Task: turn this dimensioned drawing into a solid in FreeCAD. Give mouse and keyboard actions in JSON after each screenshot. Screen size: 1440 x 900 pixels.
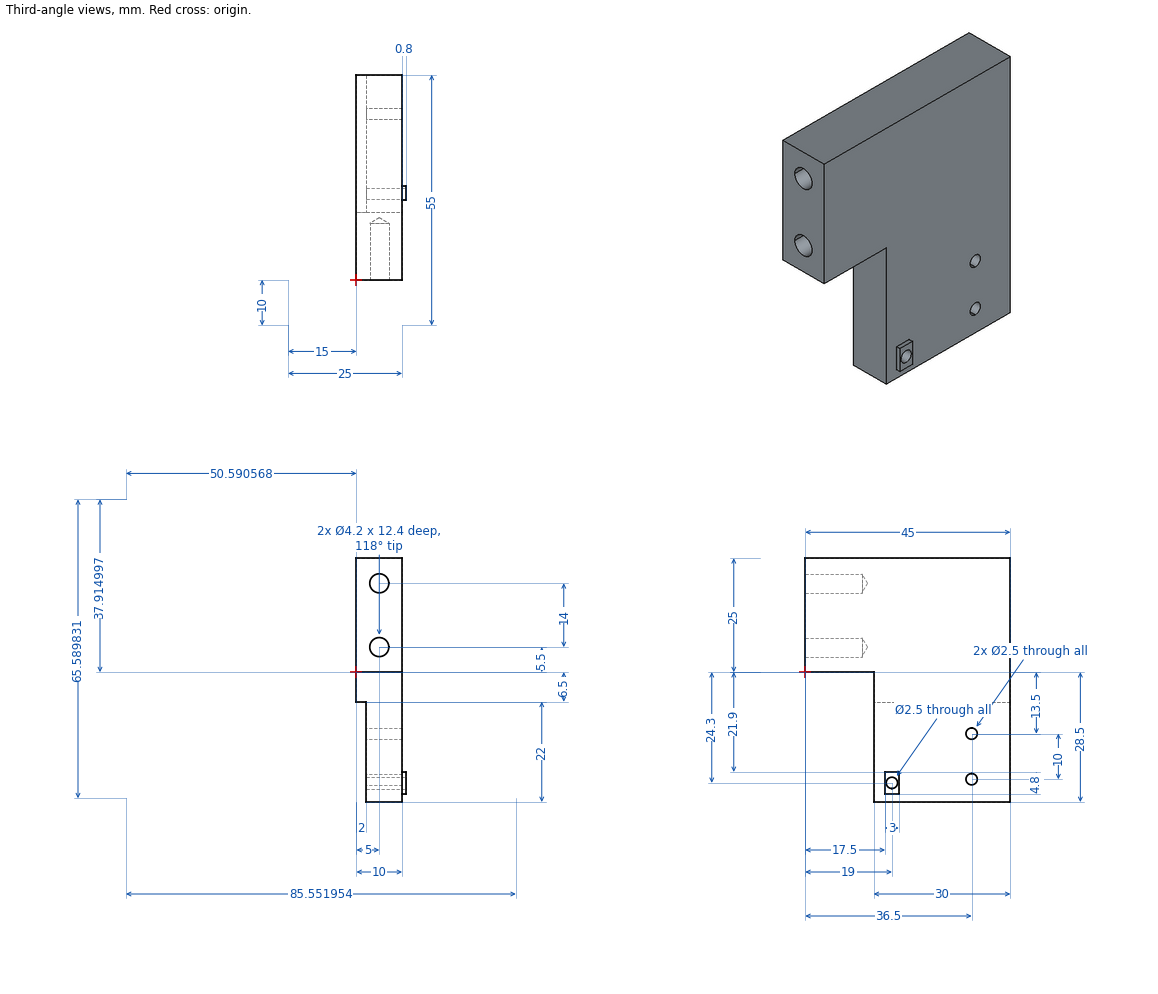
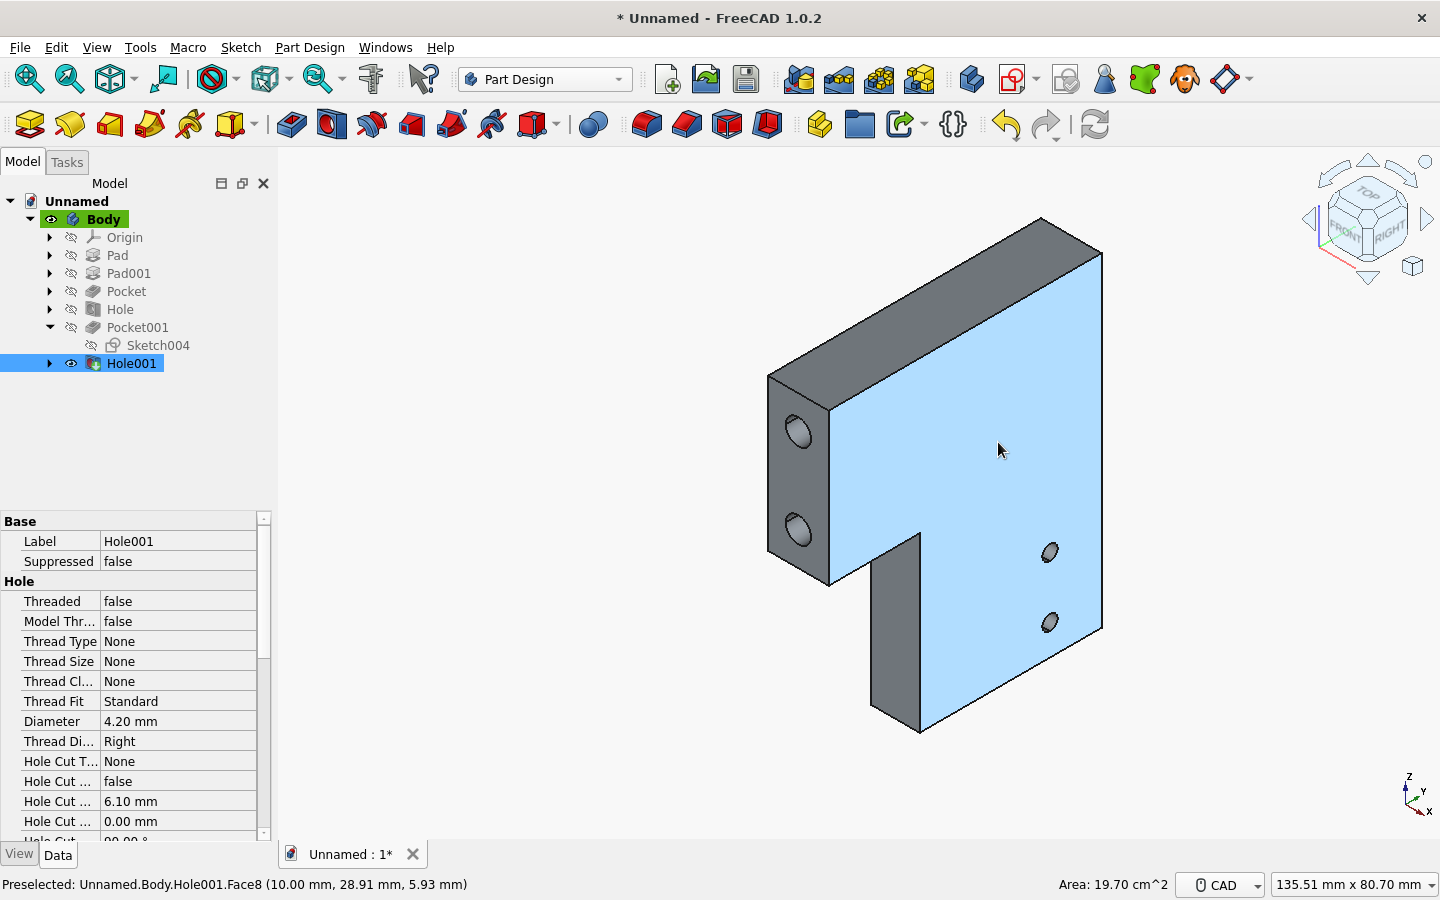
{"action": "left_click", "coordinate": [1012, 80]}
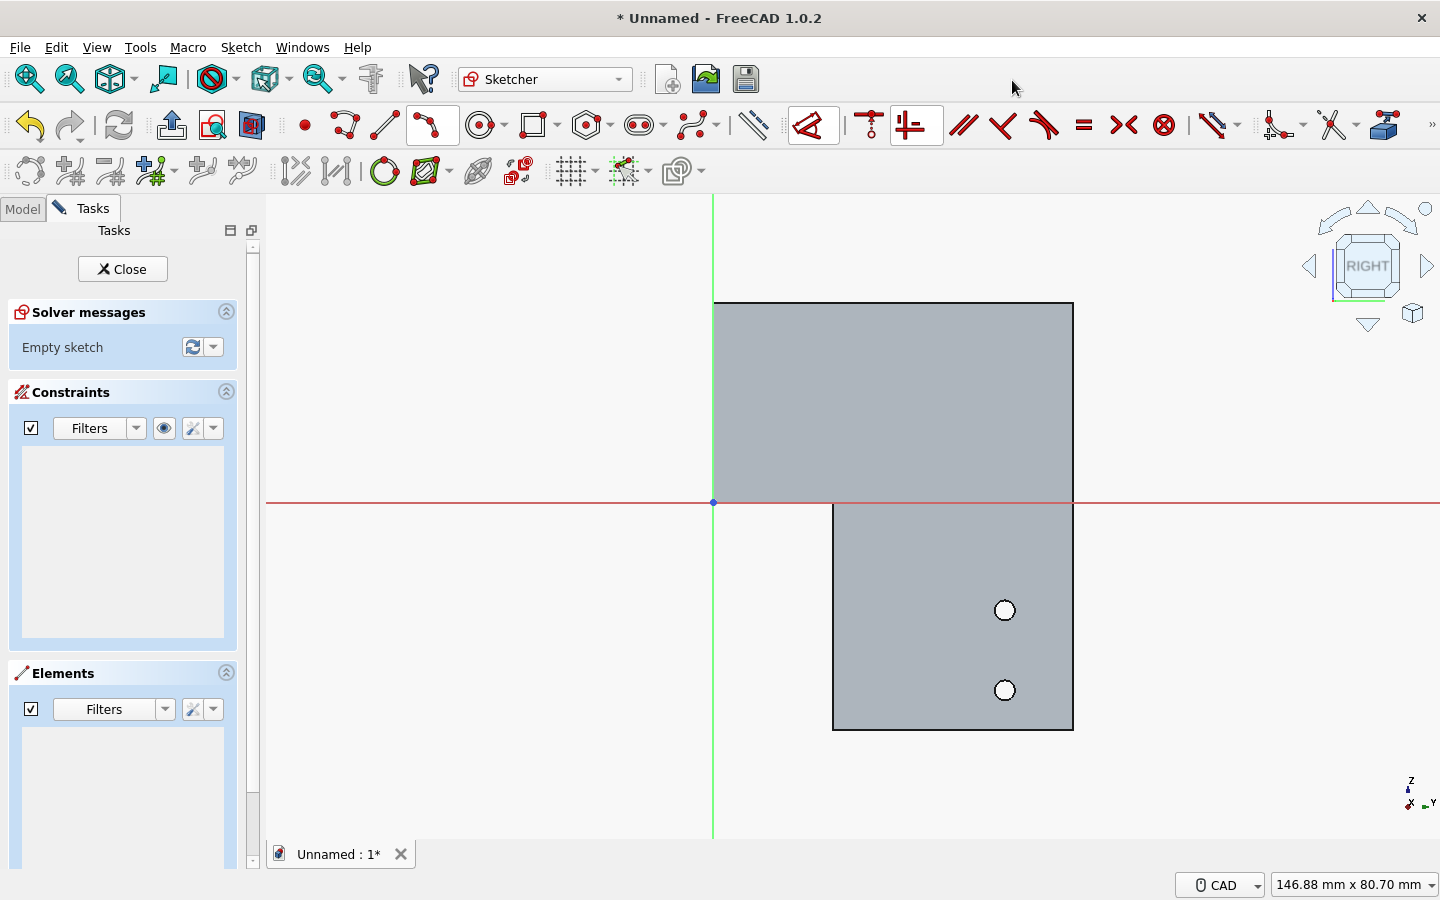
{"action": "scroll", "coordinate": [873, 715], "scroll_direction": "up", "scroll_amount": 12}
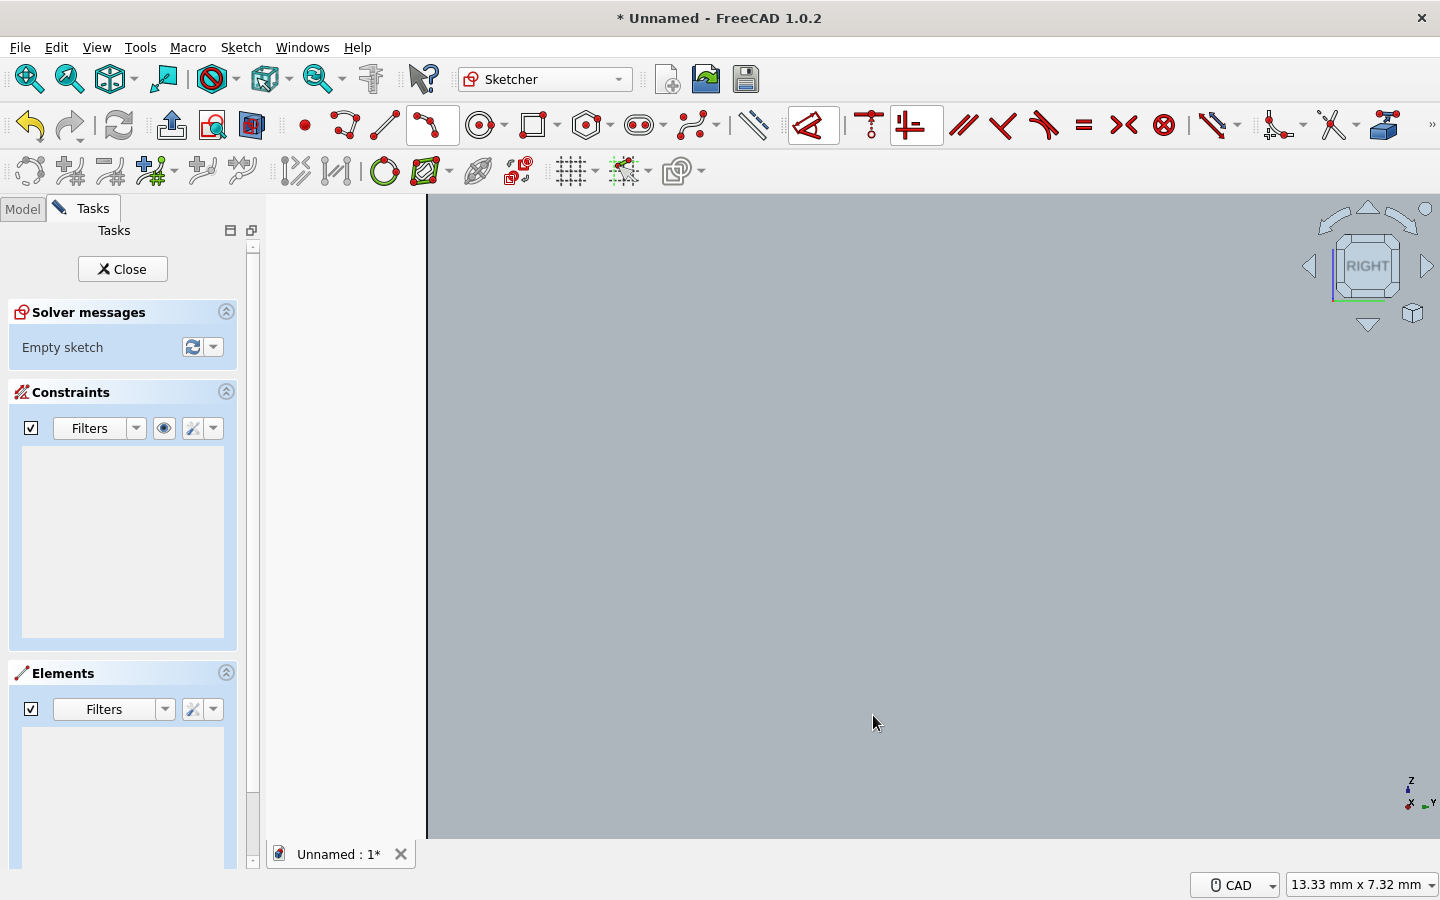
{"action": "left_click", "coordinate": [534, 126]}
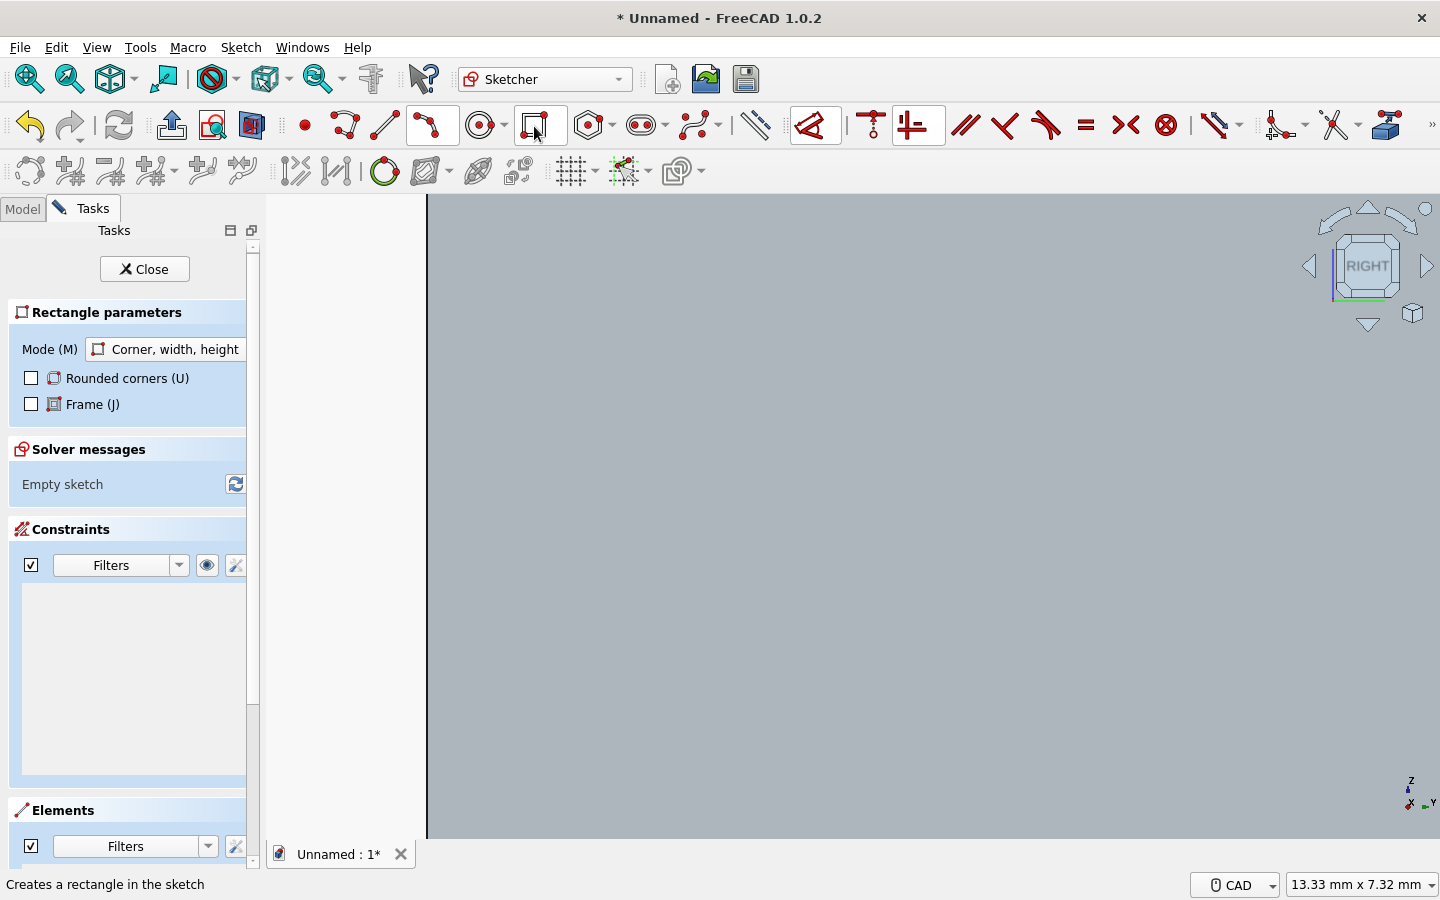
{"action": "left_click", "coordinate": [647, 294]}
{"action": "left_click", "coordinate": [912, 717]}
{"action": "key", "text": "Escape"}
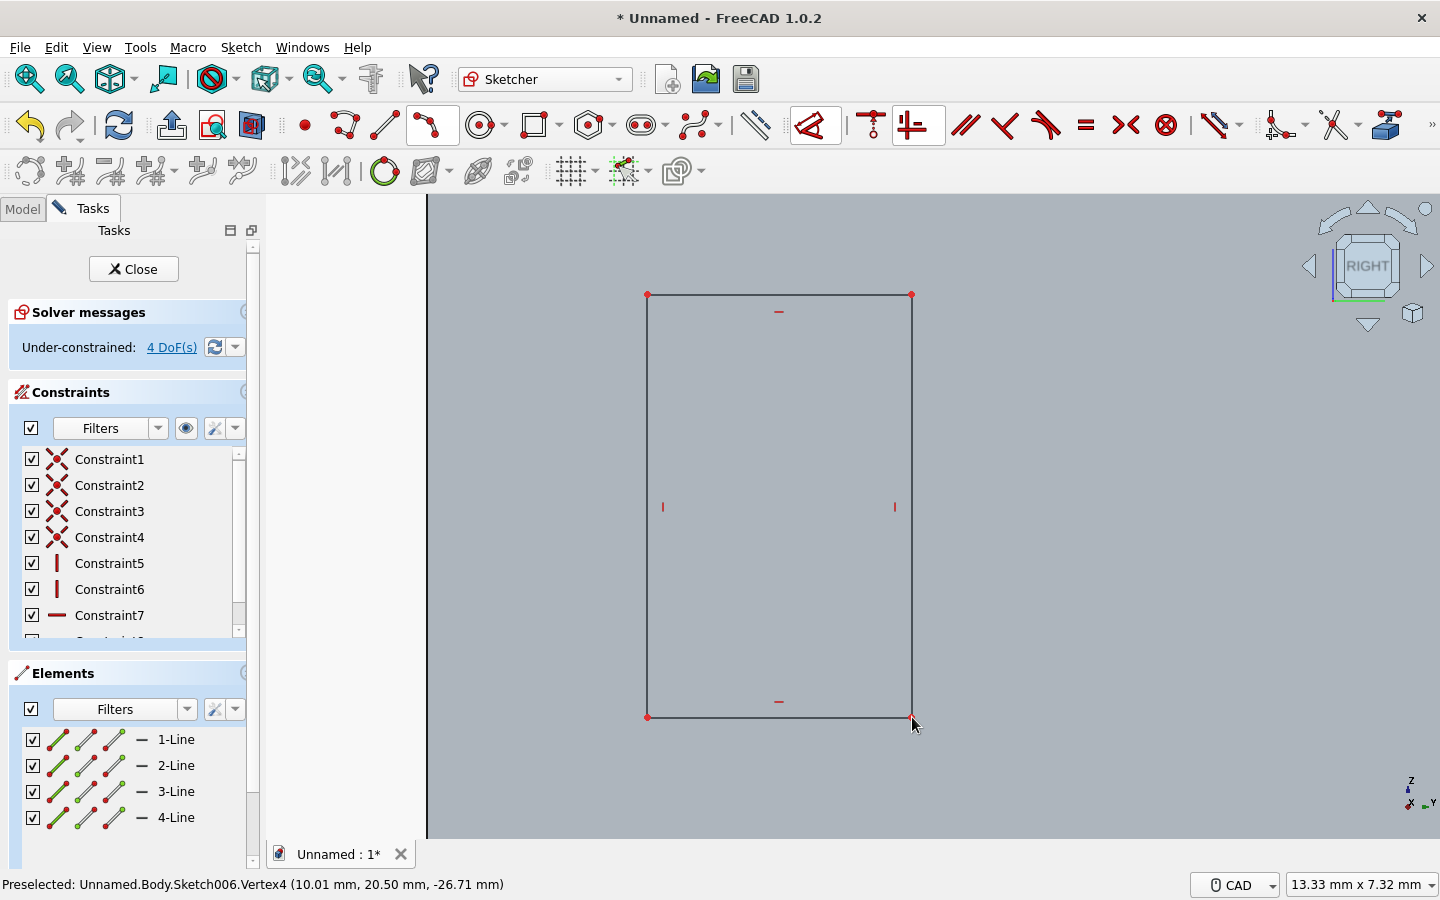
{"action": "left_click", "coordinate": [726, 718]}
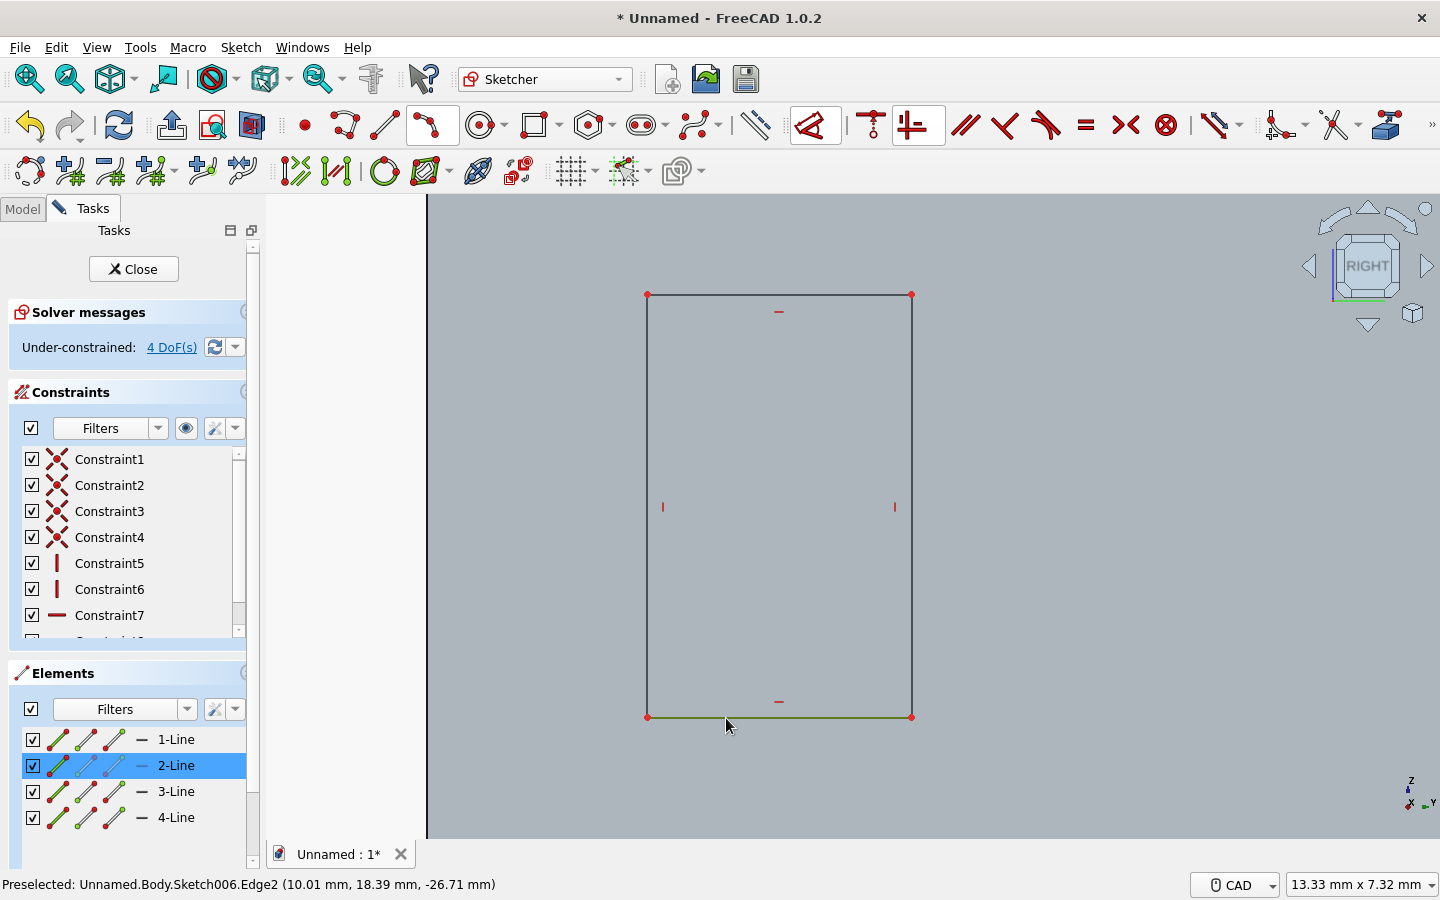
{"action": "key", "text": "l"}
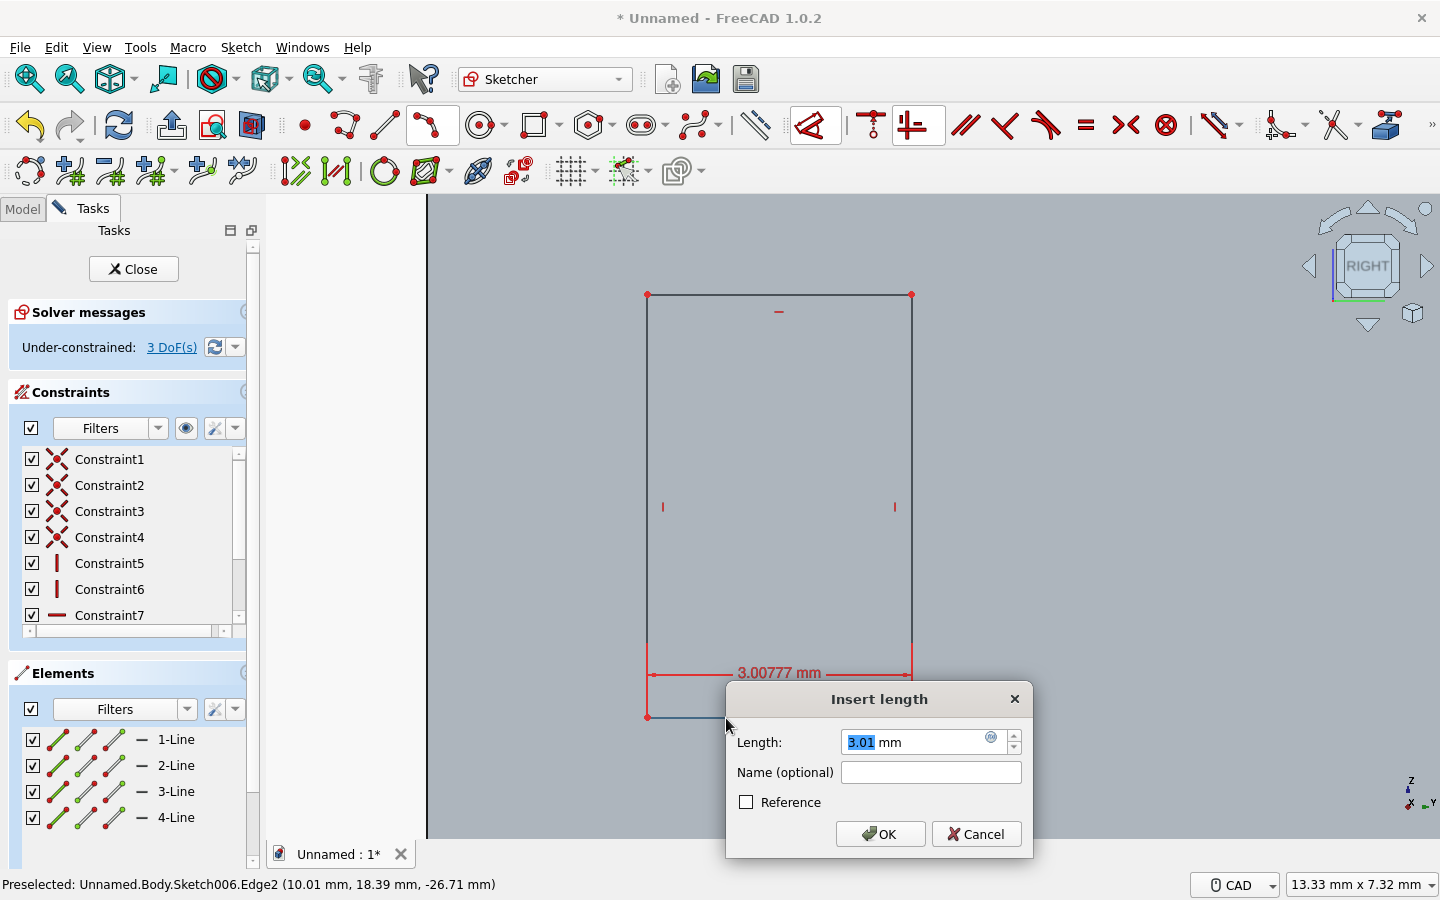
{"action": "type", "text": "3"}
{"action": "key", "text": "Return"}